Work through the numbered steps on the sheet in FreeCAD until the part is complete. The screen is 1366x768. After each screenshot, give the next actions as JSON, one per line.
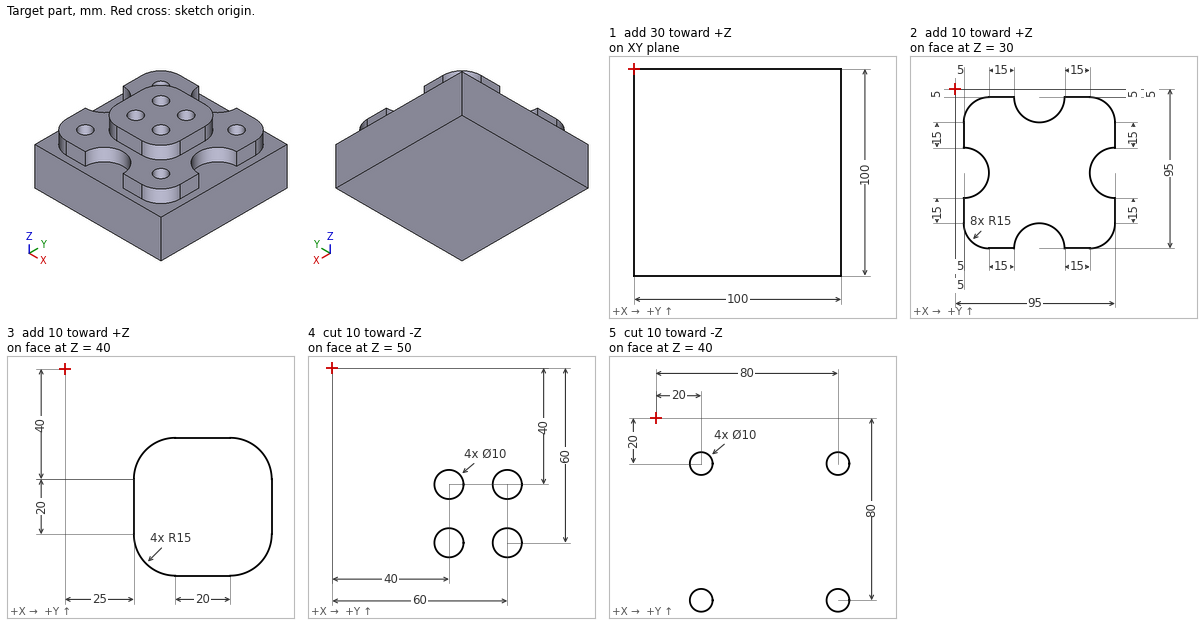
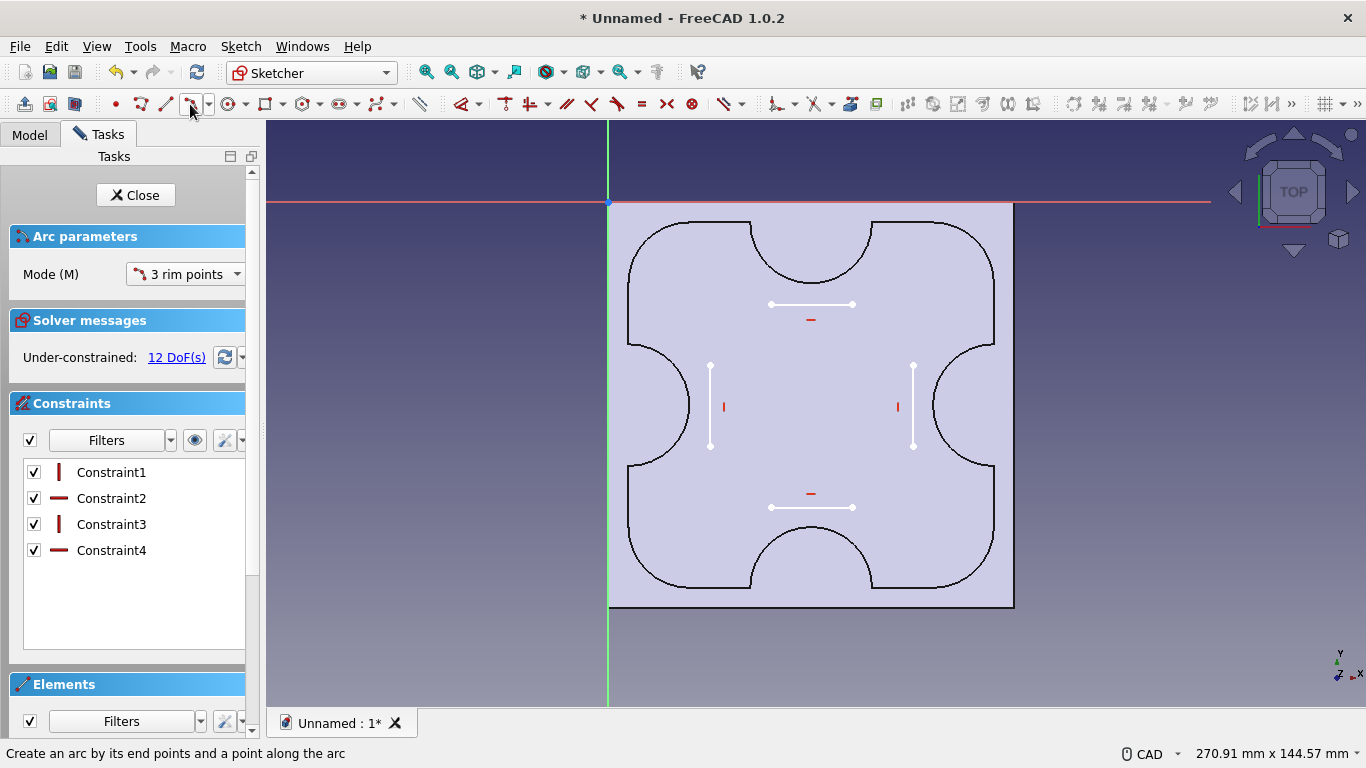
{"action": "left_click", "coordinate": [710, 447]}
{"action": "left_click", "coordinate": [771, 508]}
{"action": "left_click", "coordinate": [728, 489]}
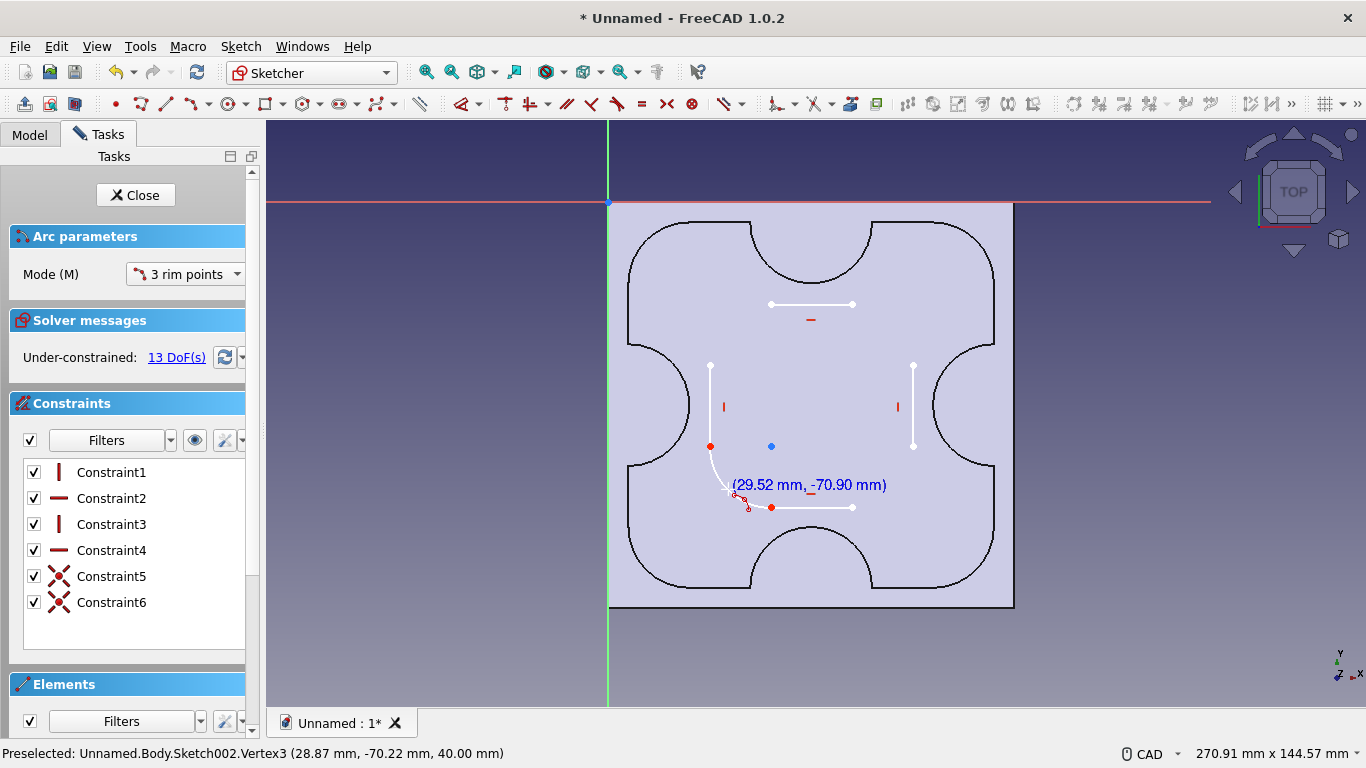
{"action": "left_click", "coordinate": [852, 508]}
{"action": "left_click", "coordinate": [913, 447]}
{"action": "left_click", "coordinate": [895, 489]}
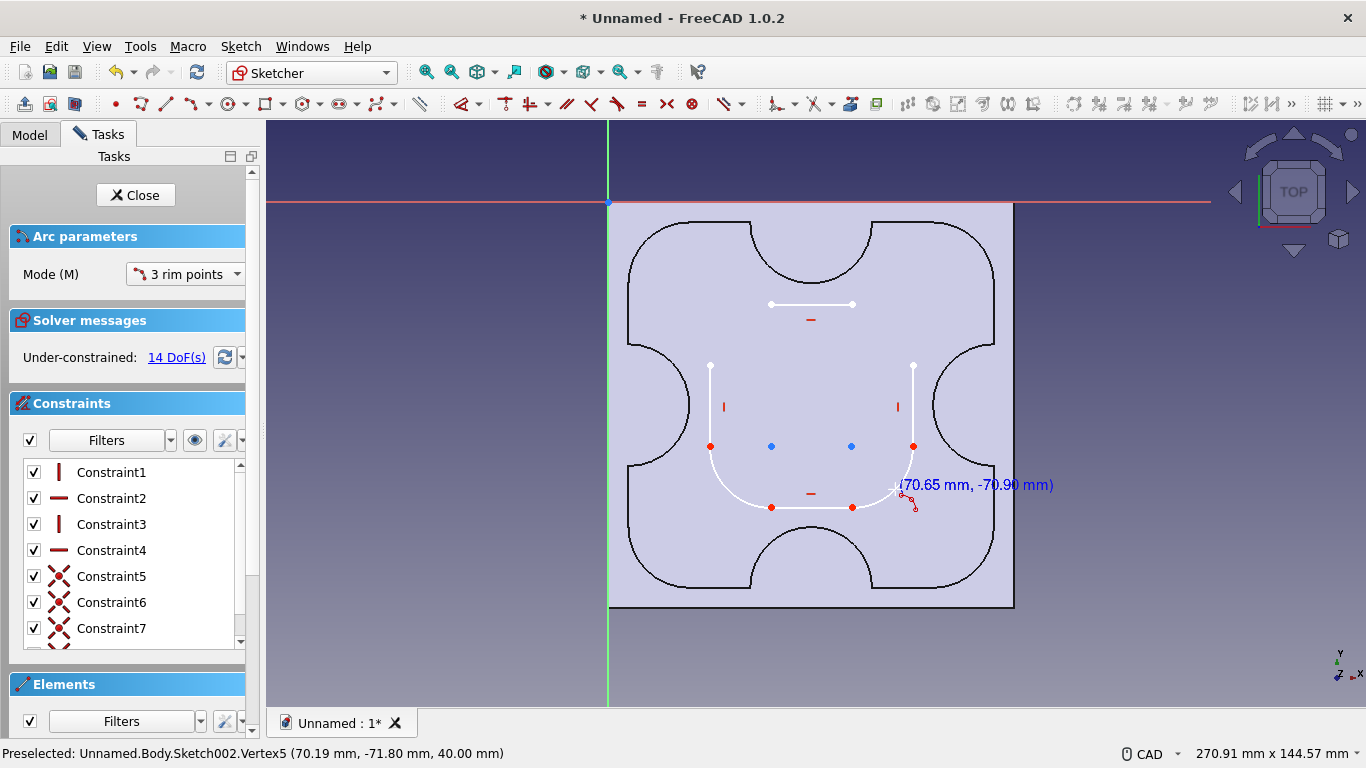
{"action": "left_click", "coordinate": [913, 366]}
{"action": "left_click", "coordinate": [852, 305]}
{"action": "left_click", "coordinate": [895, 321]}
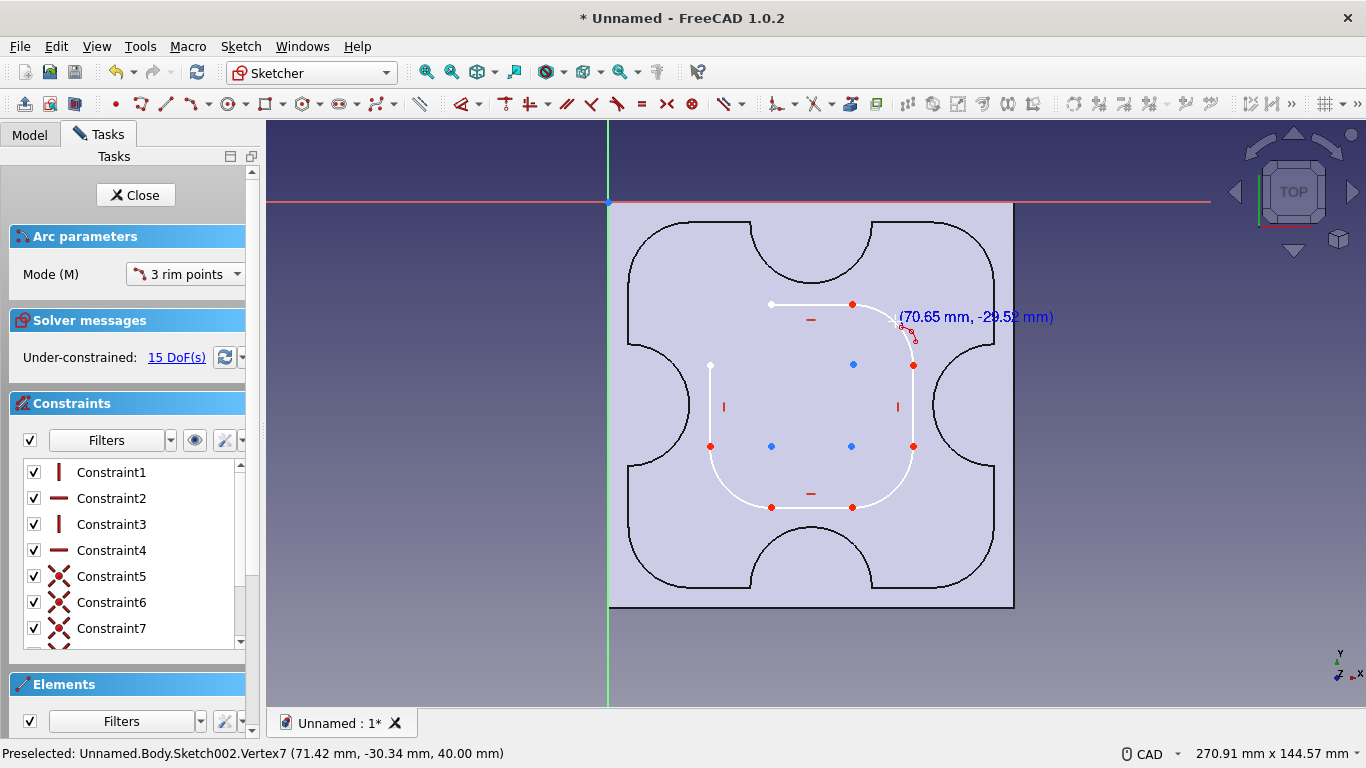
{"action": "left_click", "coordinate": [771, 305]}
{"action": "left_click", "coordinate": [710, 366]}
{"action": "left_click", "coordinate": [728, 321]}
{"action": "key", "text": "Escape"}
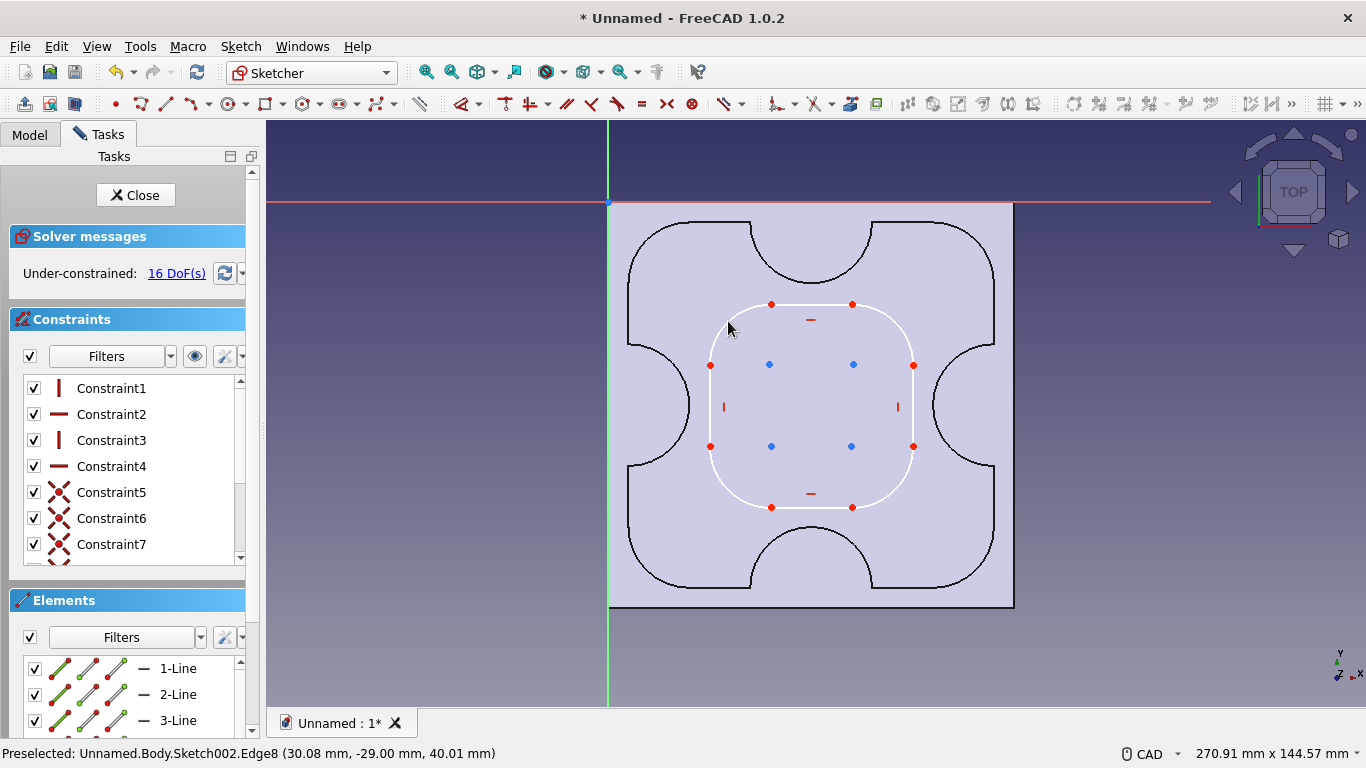
{"action": "left_click", "coordinate": [710, 390]}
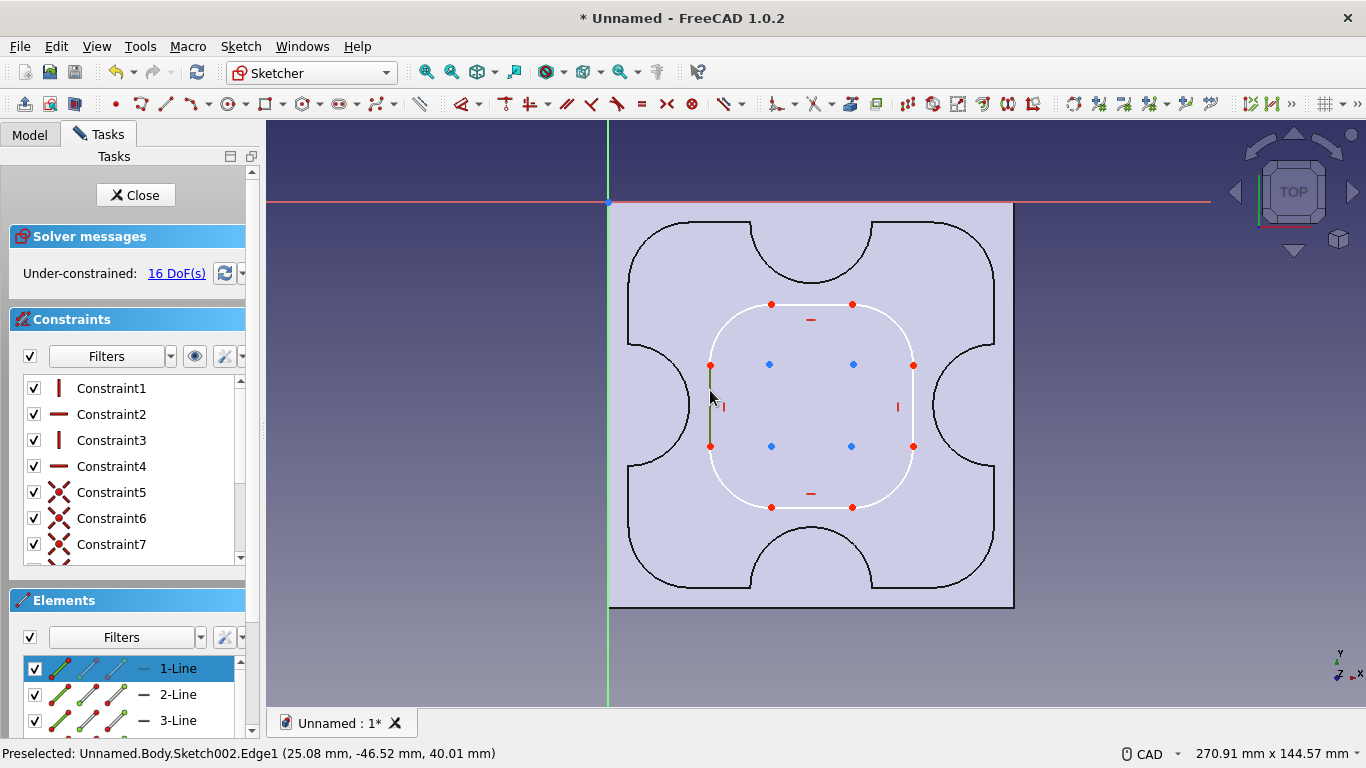
{"action": "left_click", "coordinate": [717, 475]}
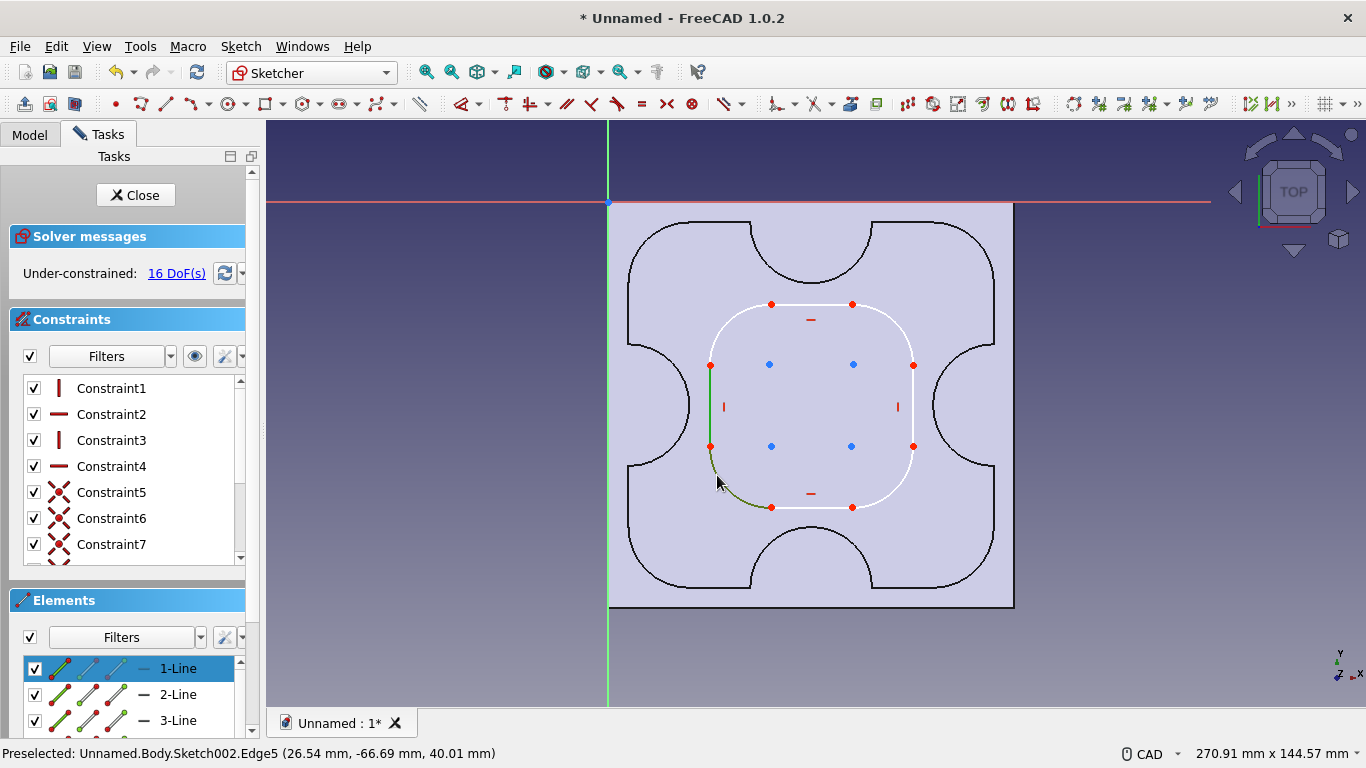
{"action": "key", "text": "t"}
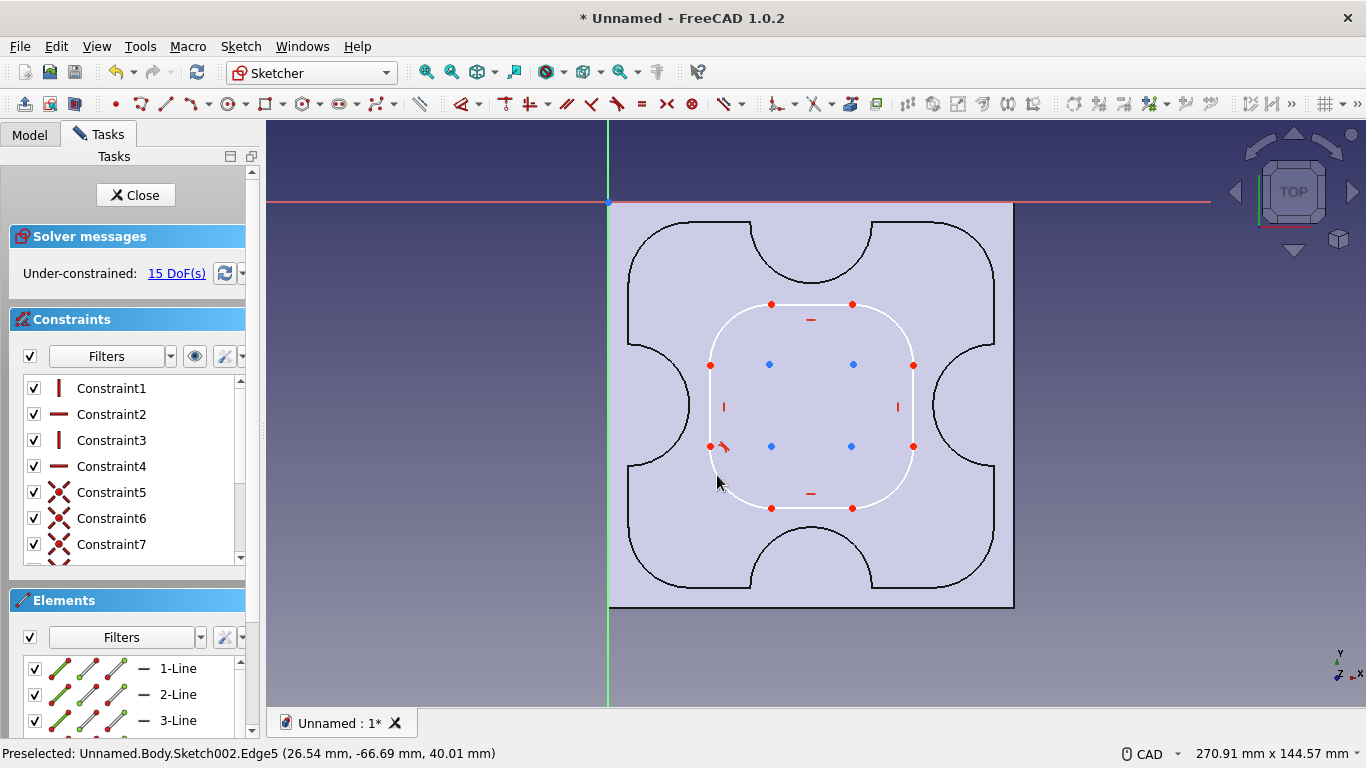
{"action": "left_click", "coordinate": [710, 390]}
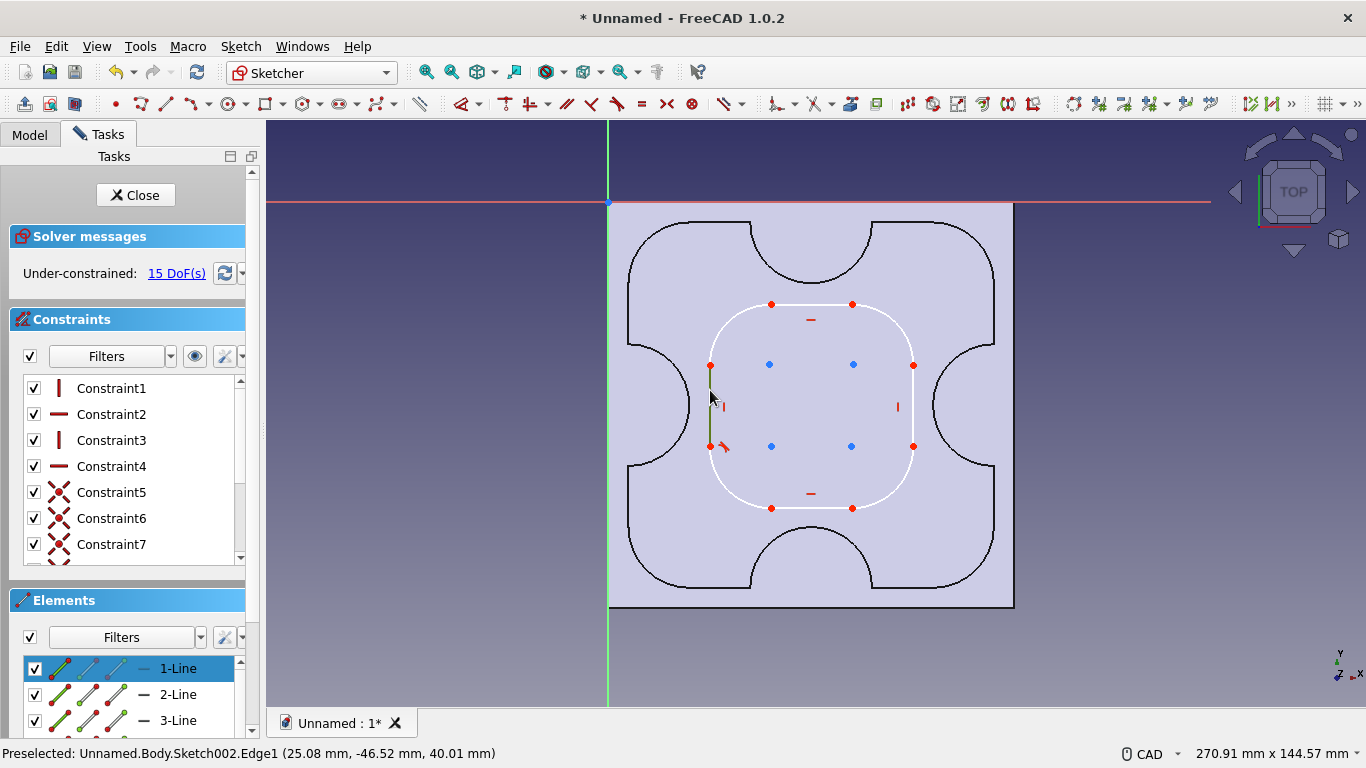
{"action": "left_click", "coordinate": [743, 311]}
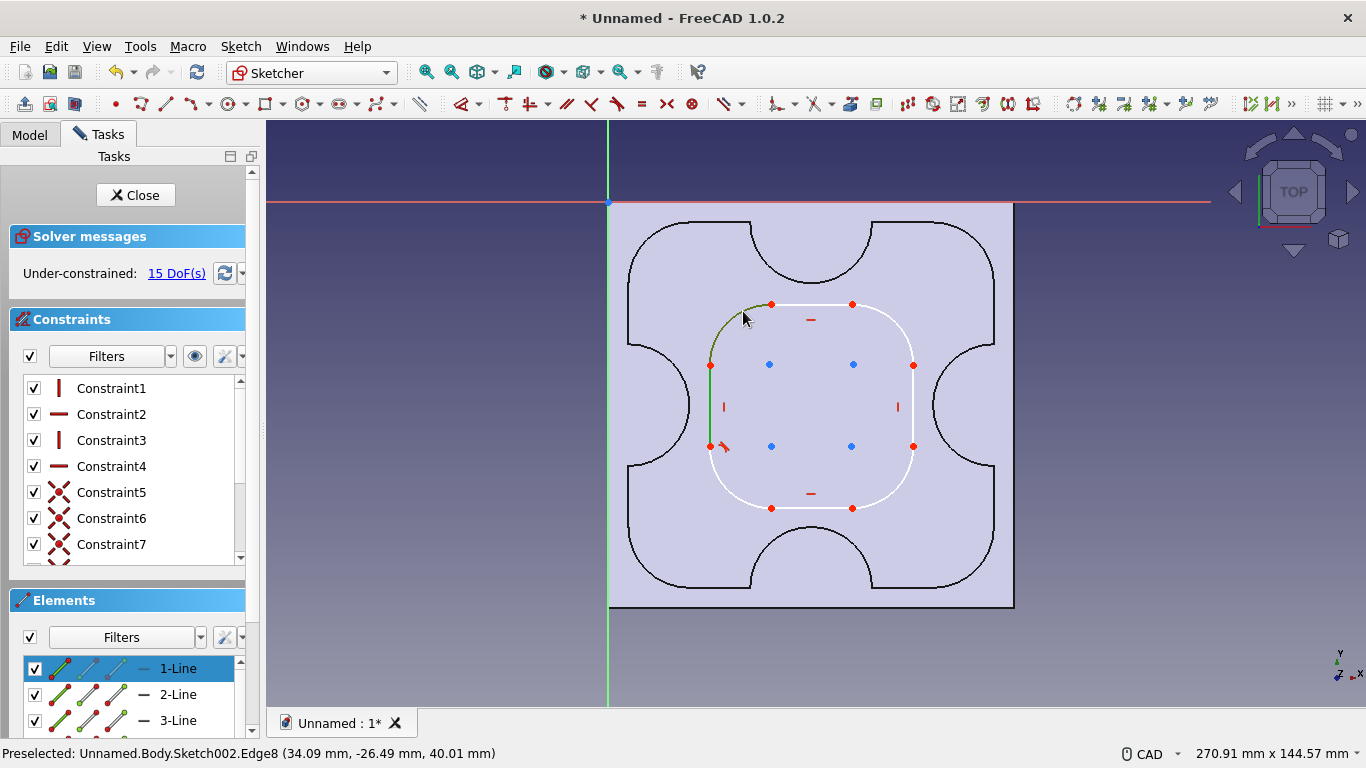
{"action": "left_click", "coordinate": [617, 104]}